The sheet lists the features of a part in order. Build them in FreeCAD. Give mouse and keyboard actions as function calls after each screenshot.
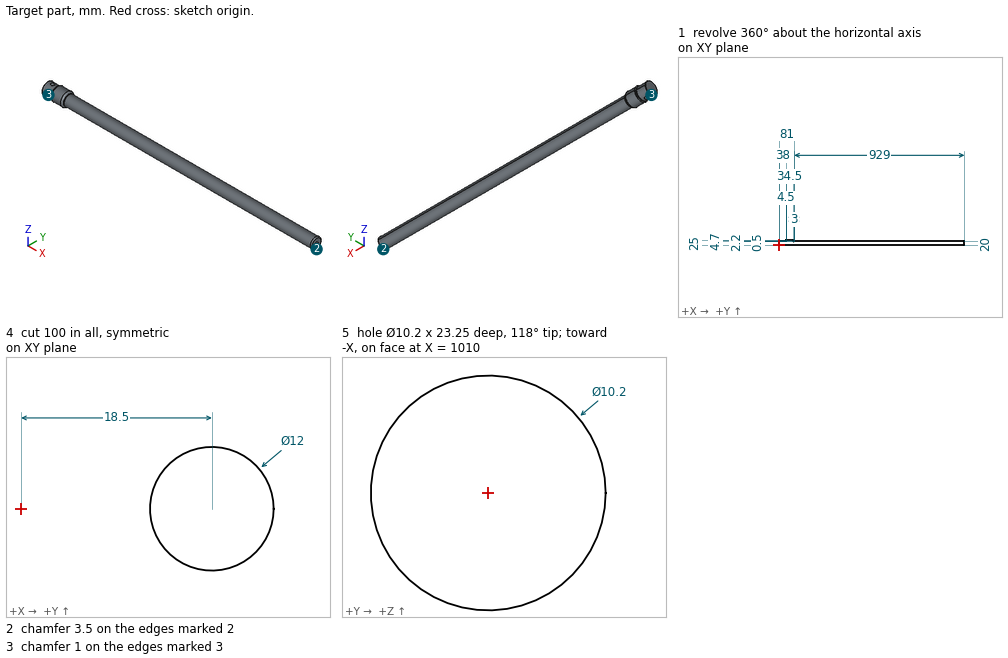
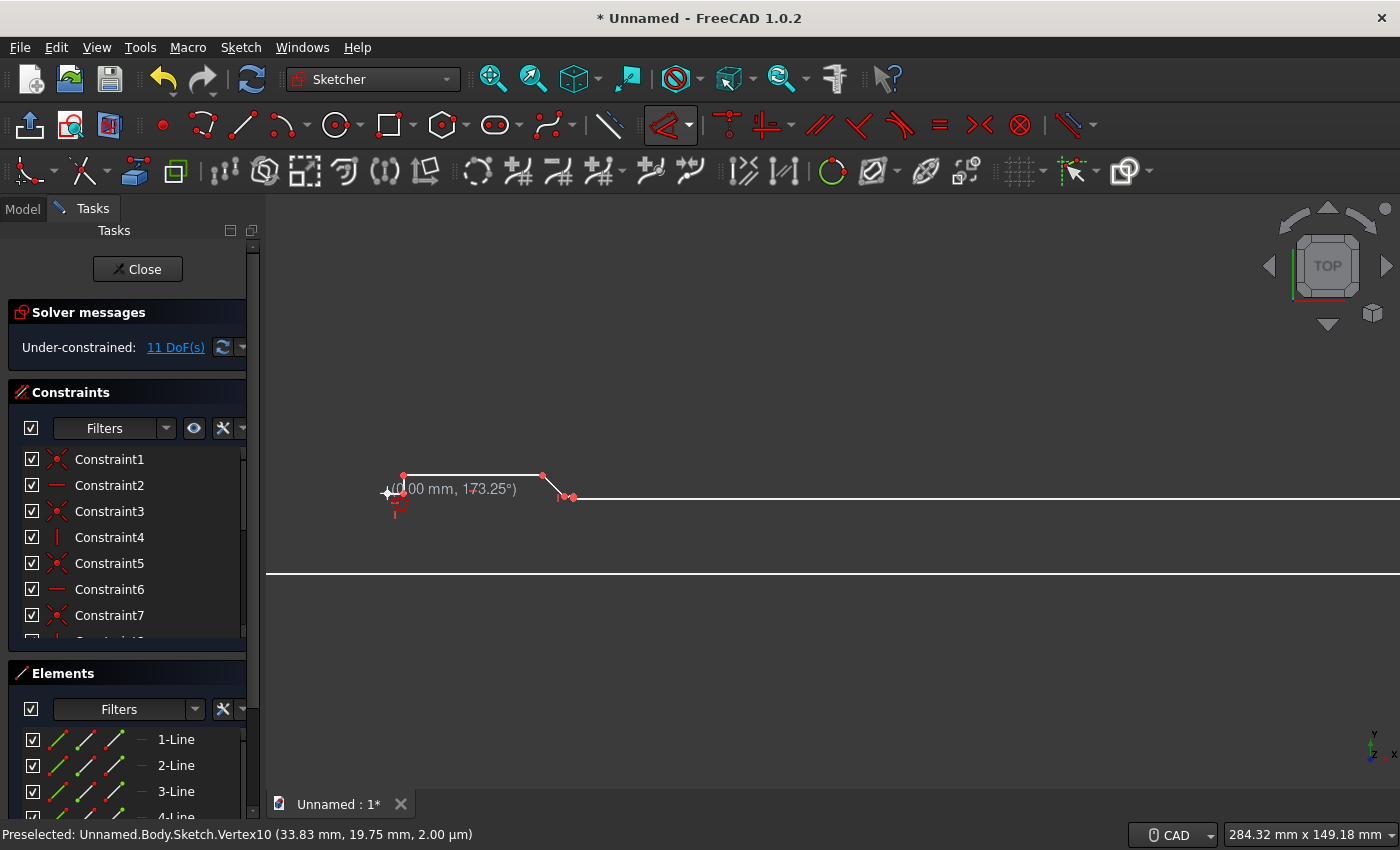
scroll(387, 484, up, 3)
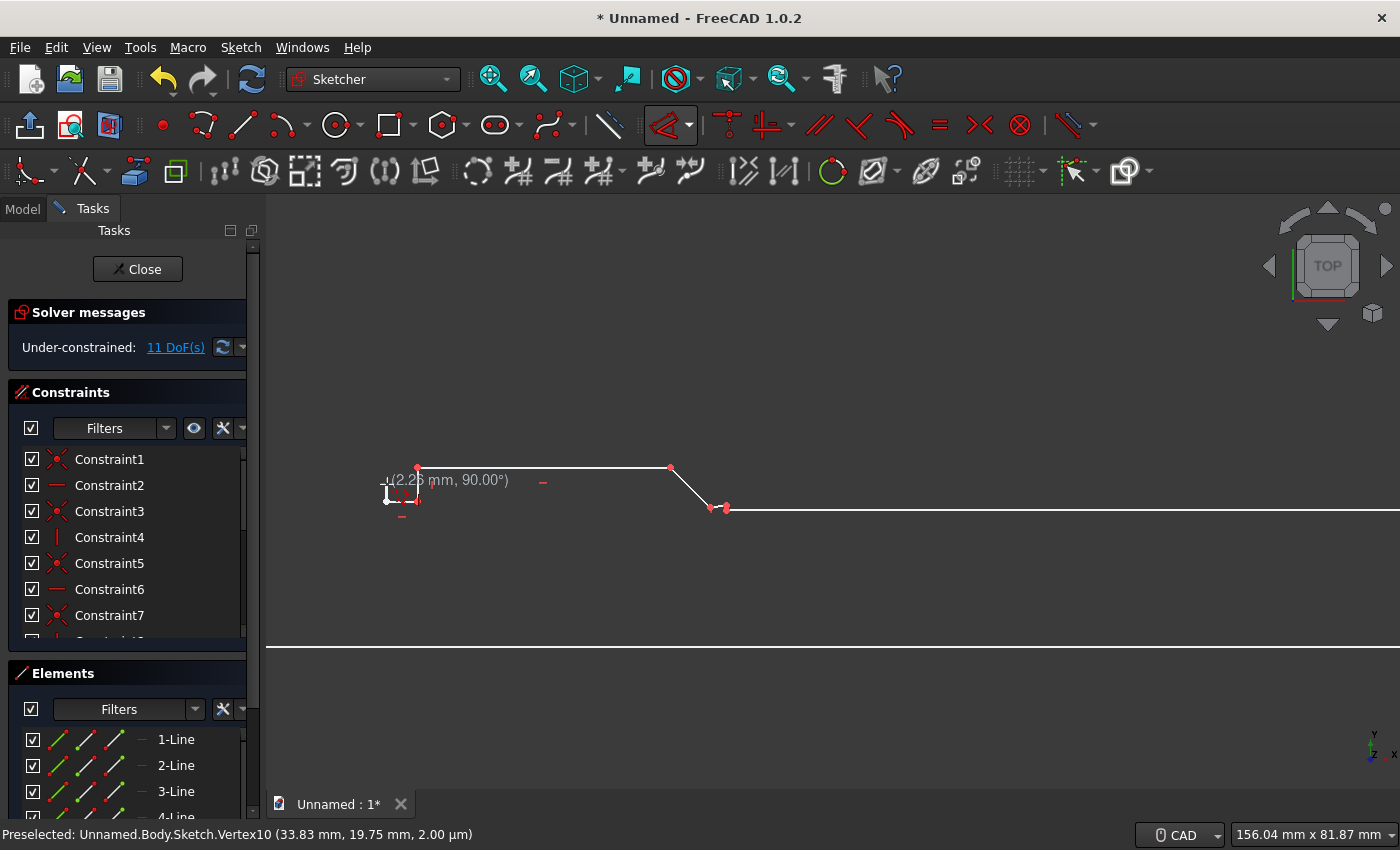
click(387, 484)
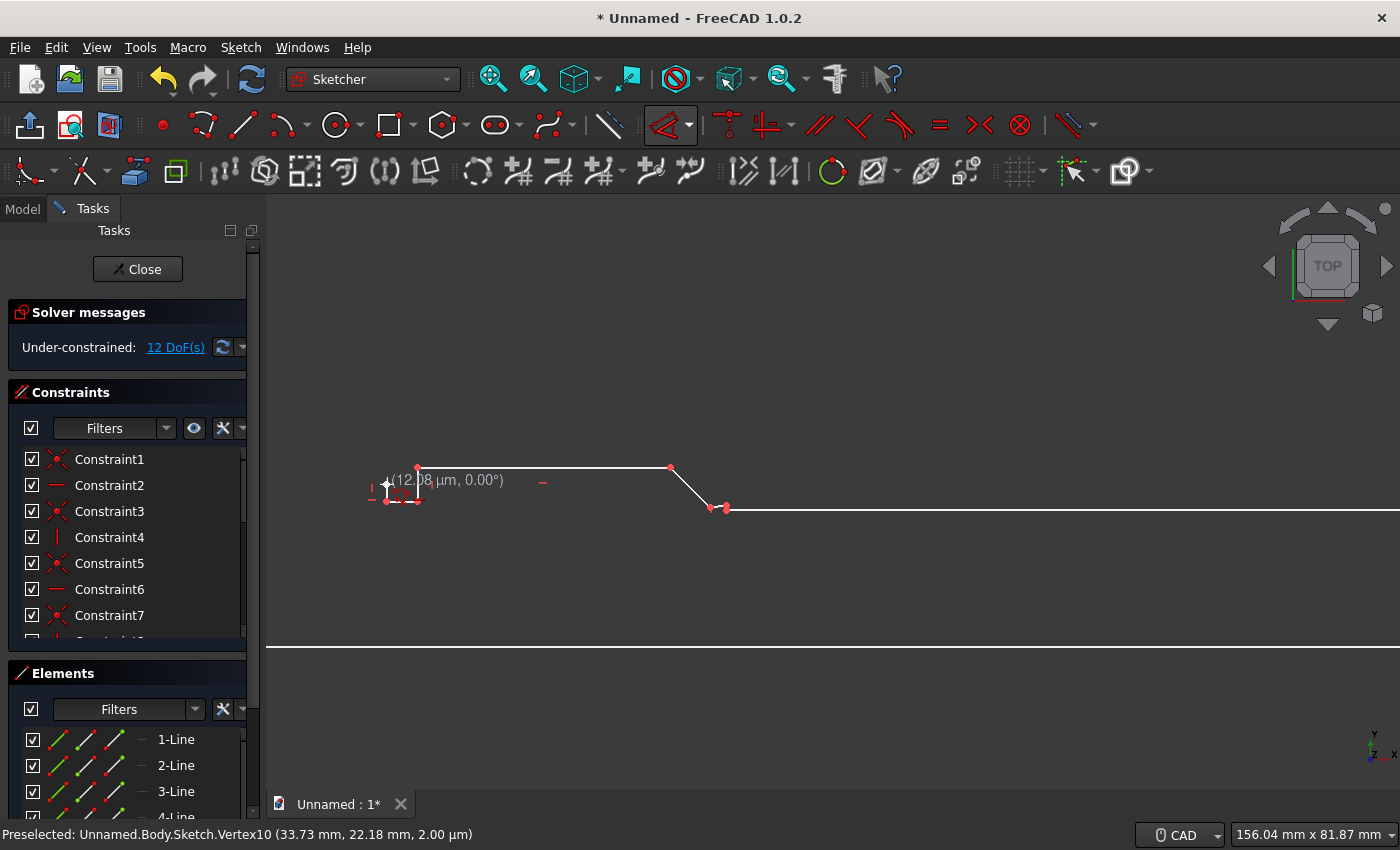
scroll(460, 485, down, 12)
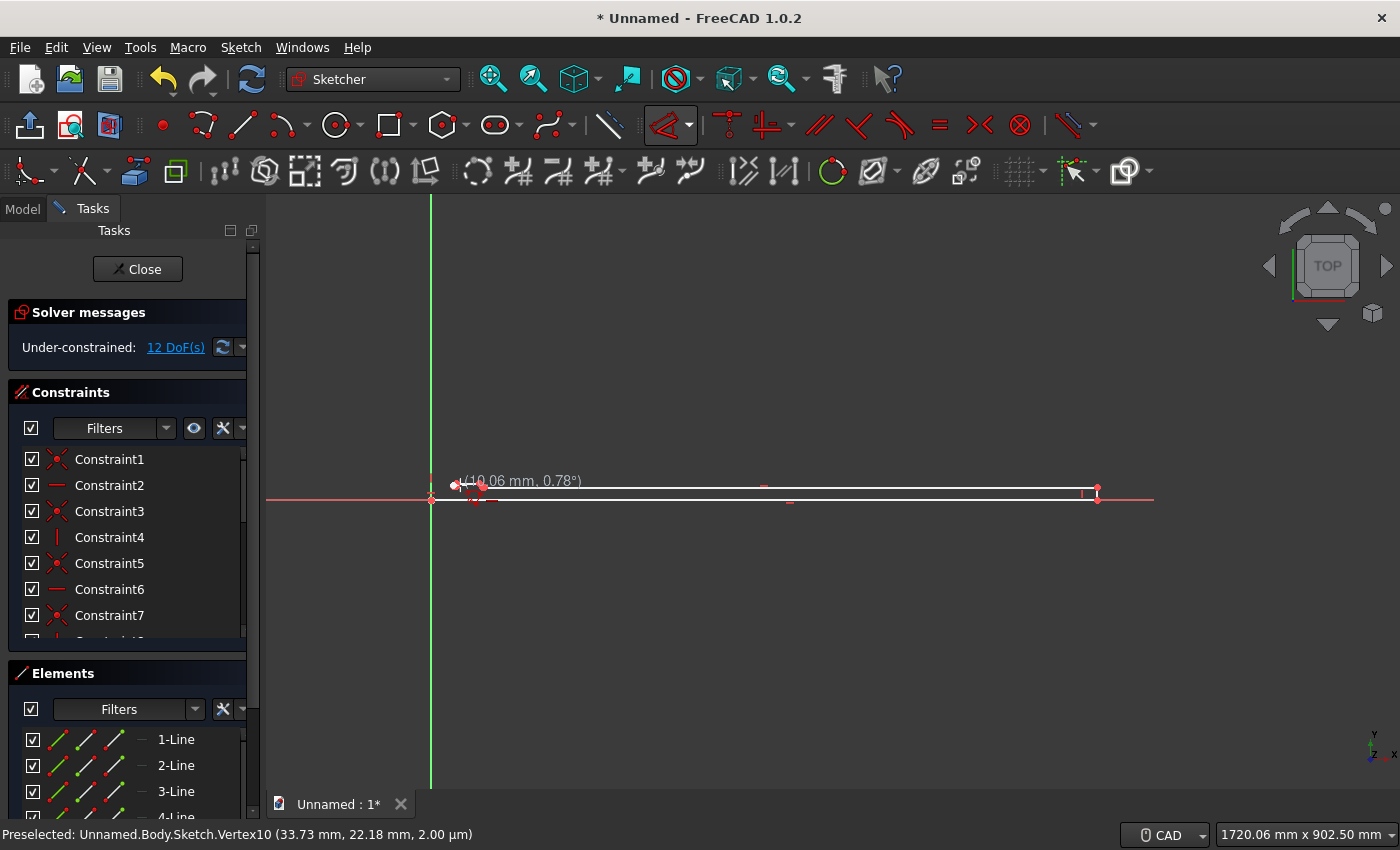
click(440, 485)
click(431, 500)
key(Escape)
key(Escape)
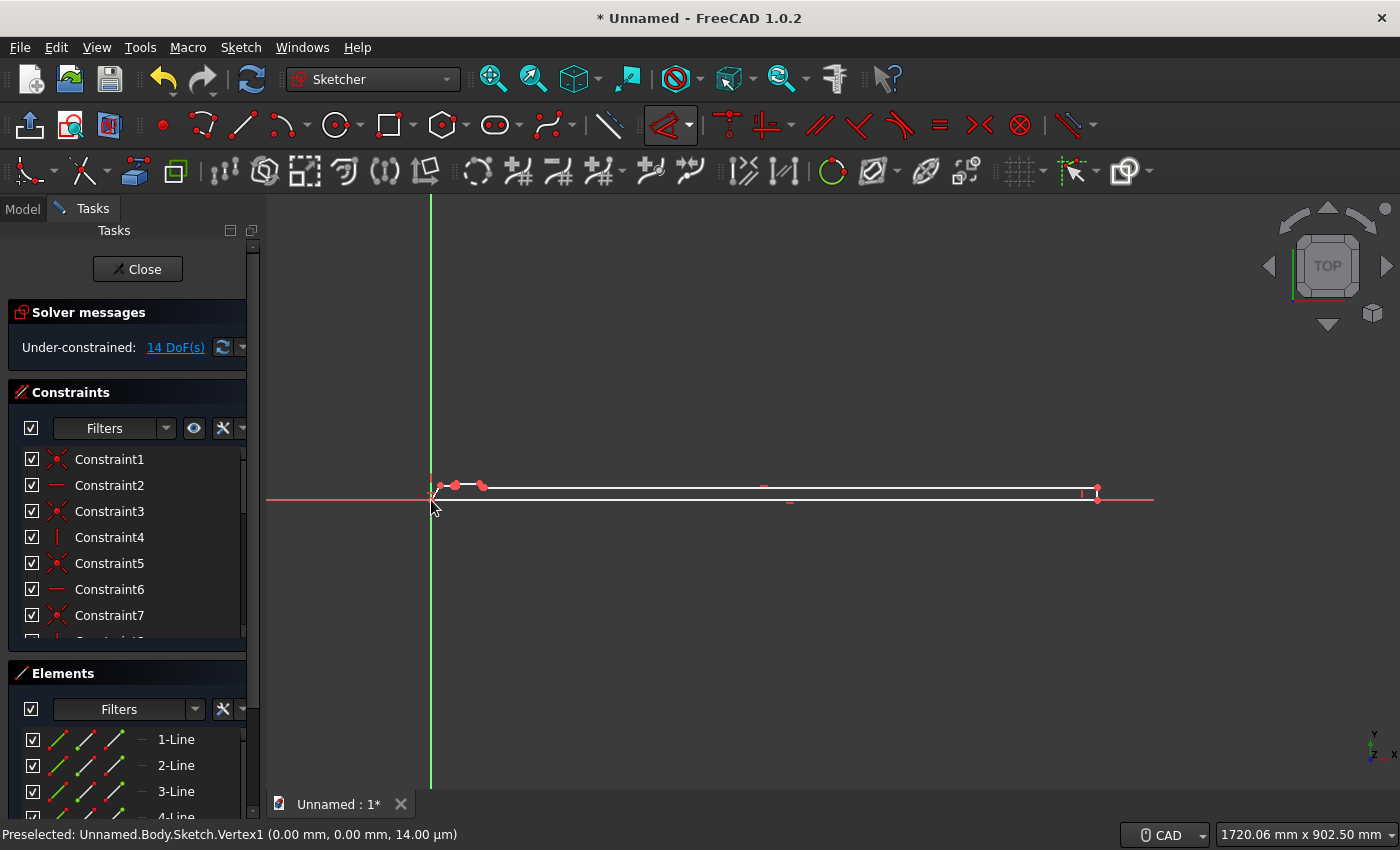
scroll(484, 487, up, 14)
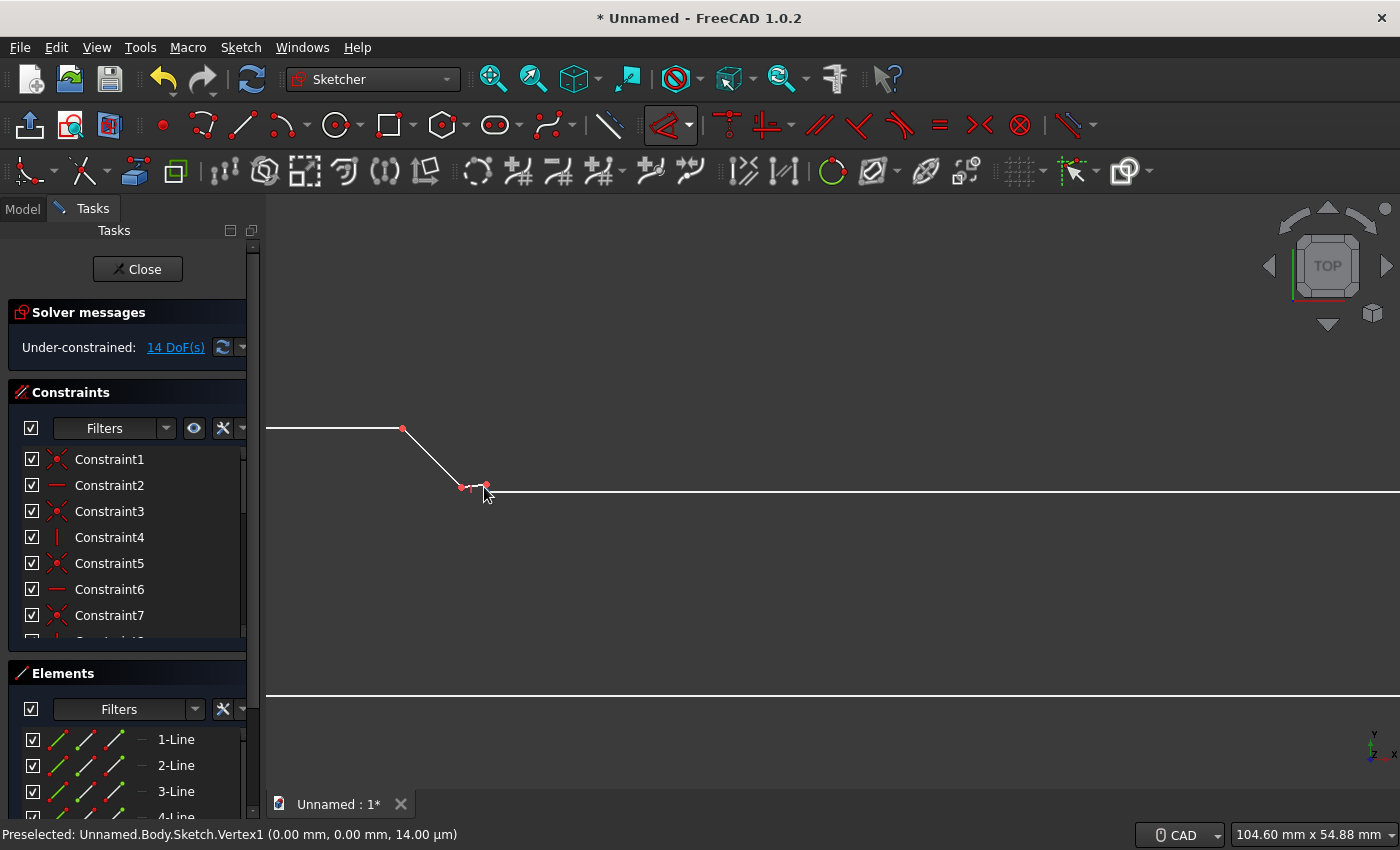
click(479, 485)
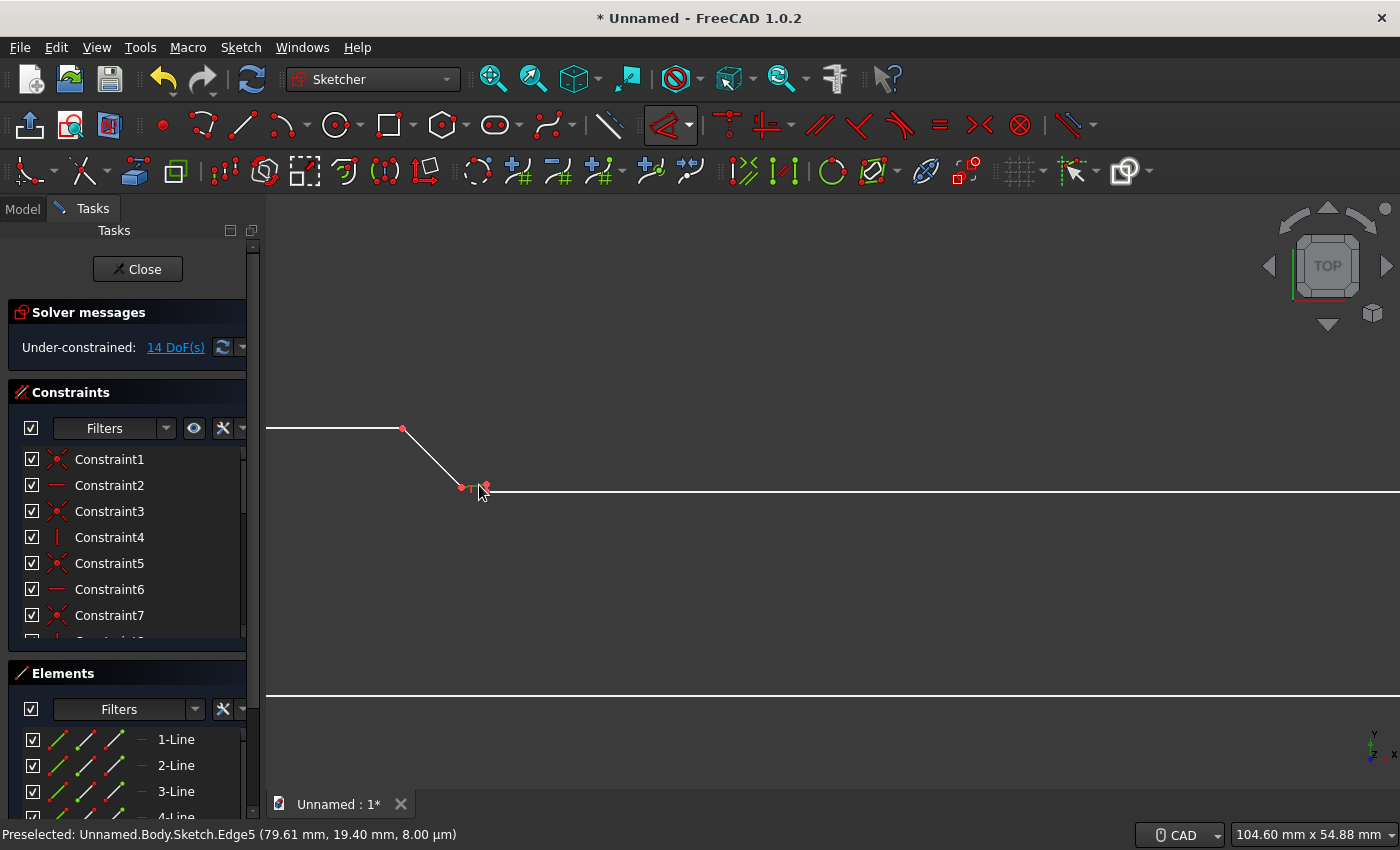
key(h)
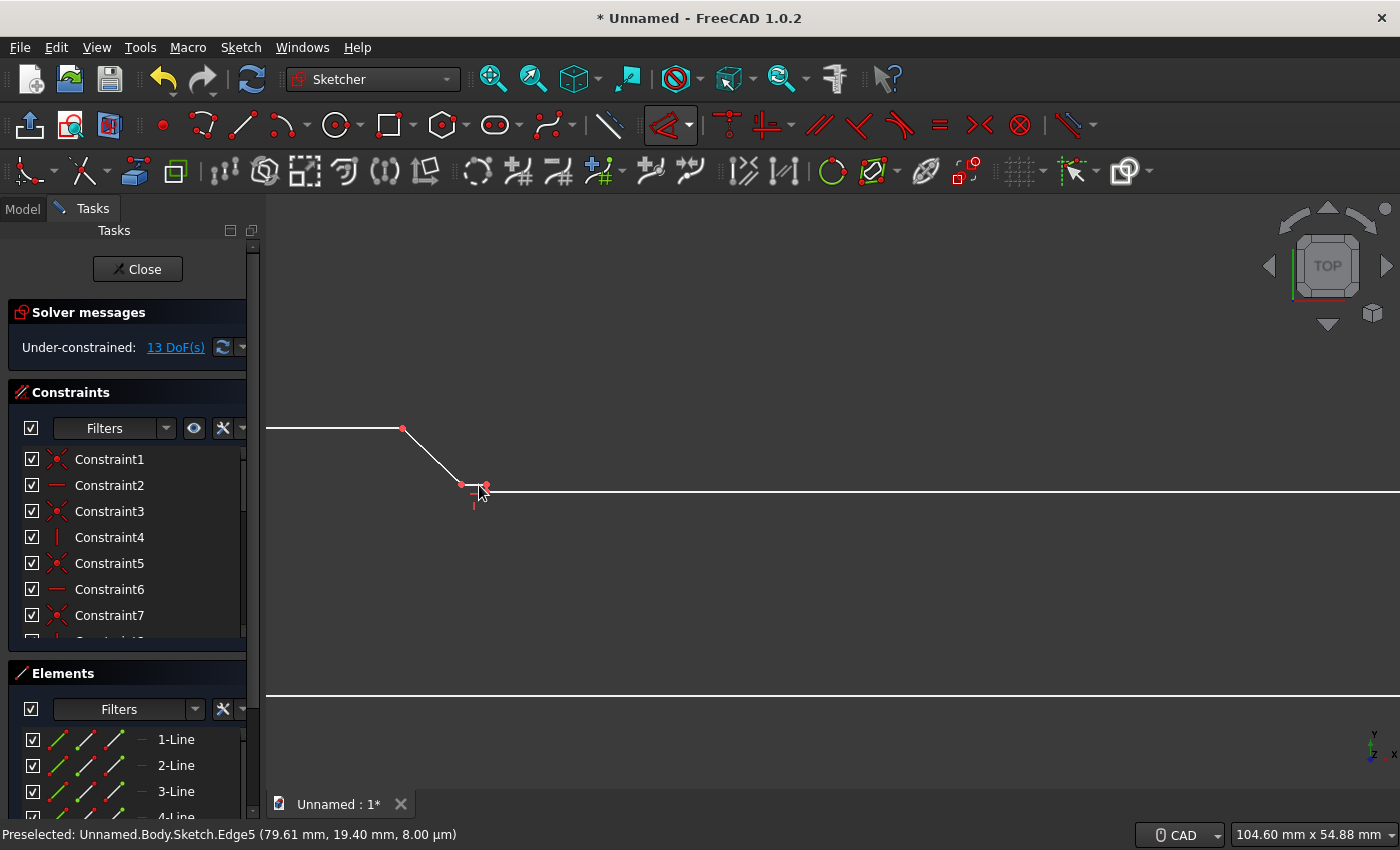
scroll(484, 487, down, 14)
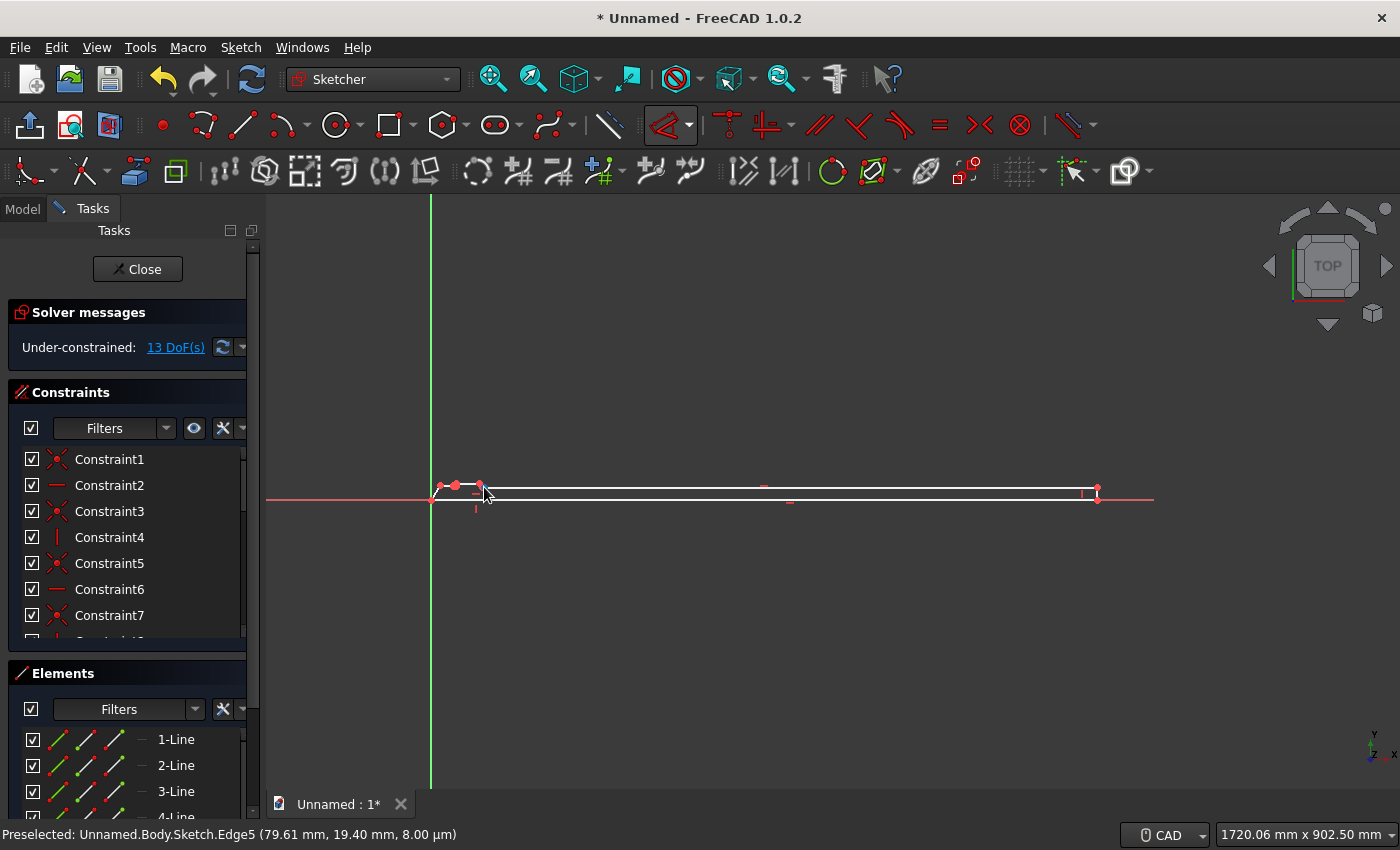
scroll(449, 486, up, 7)